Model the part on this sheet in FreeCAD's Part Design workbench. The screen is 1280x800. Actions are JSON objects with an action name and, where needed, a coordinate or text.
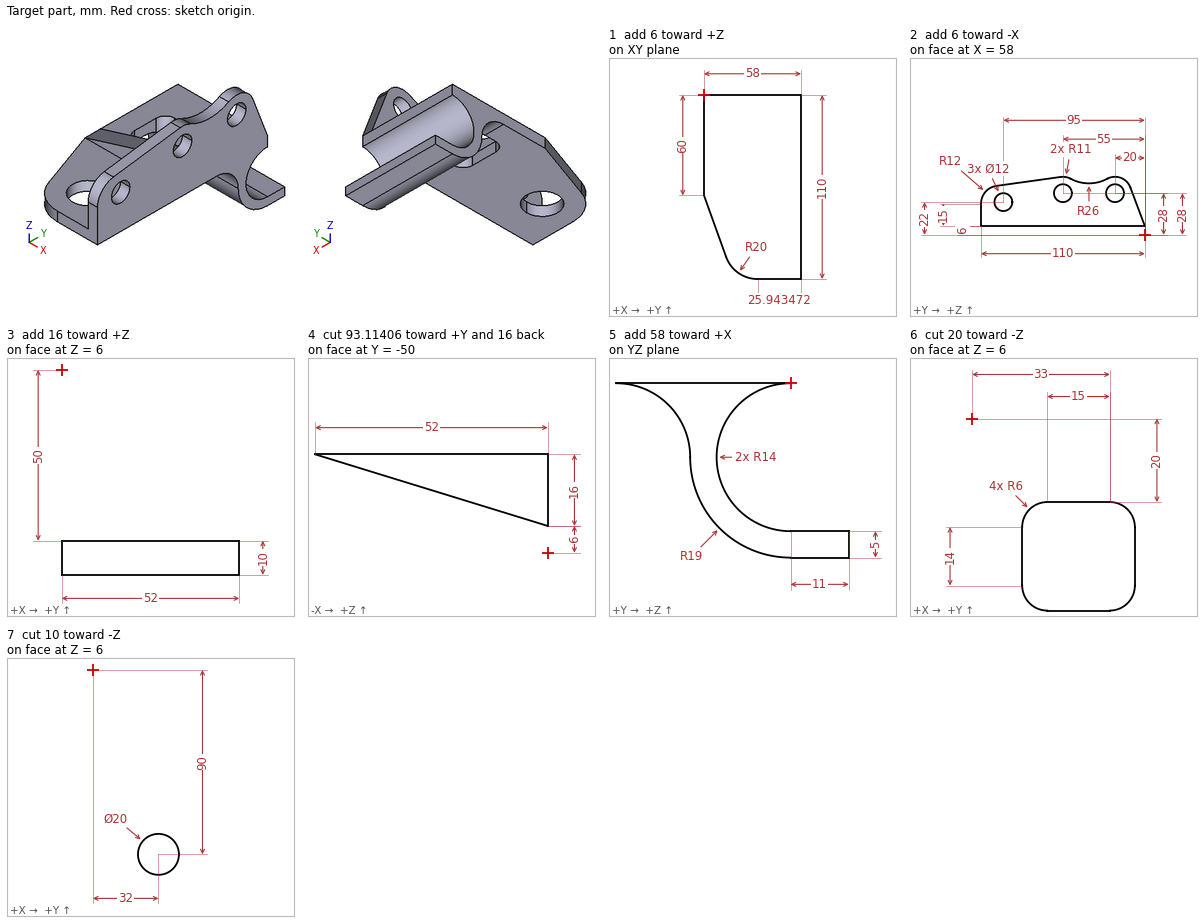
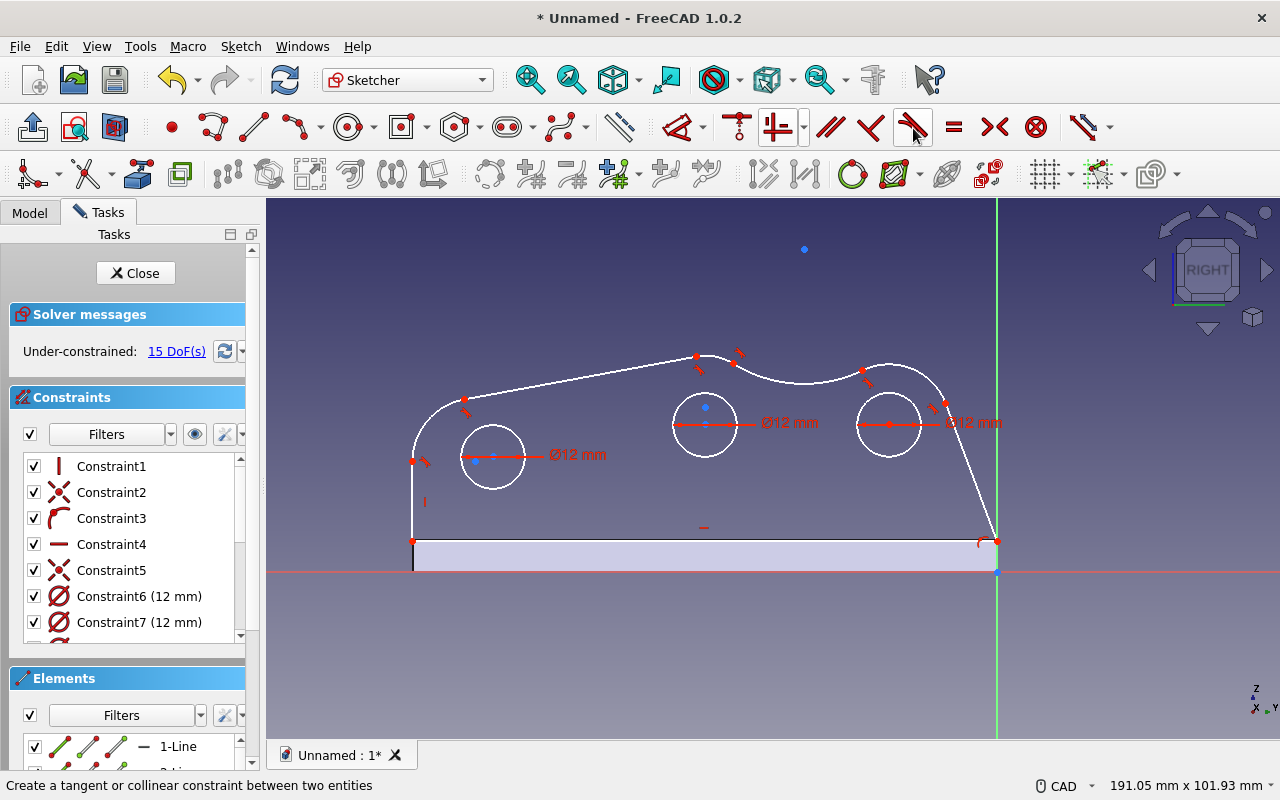
{"action": "left_click", "coordinate": [727, 402]}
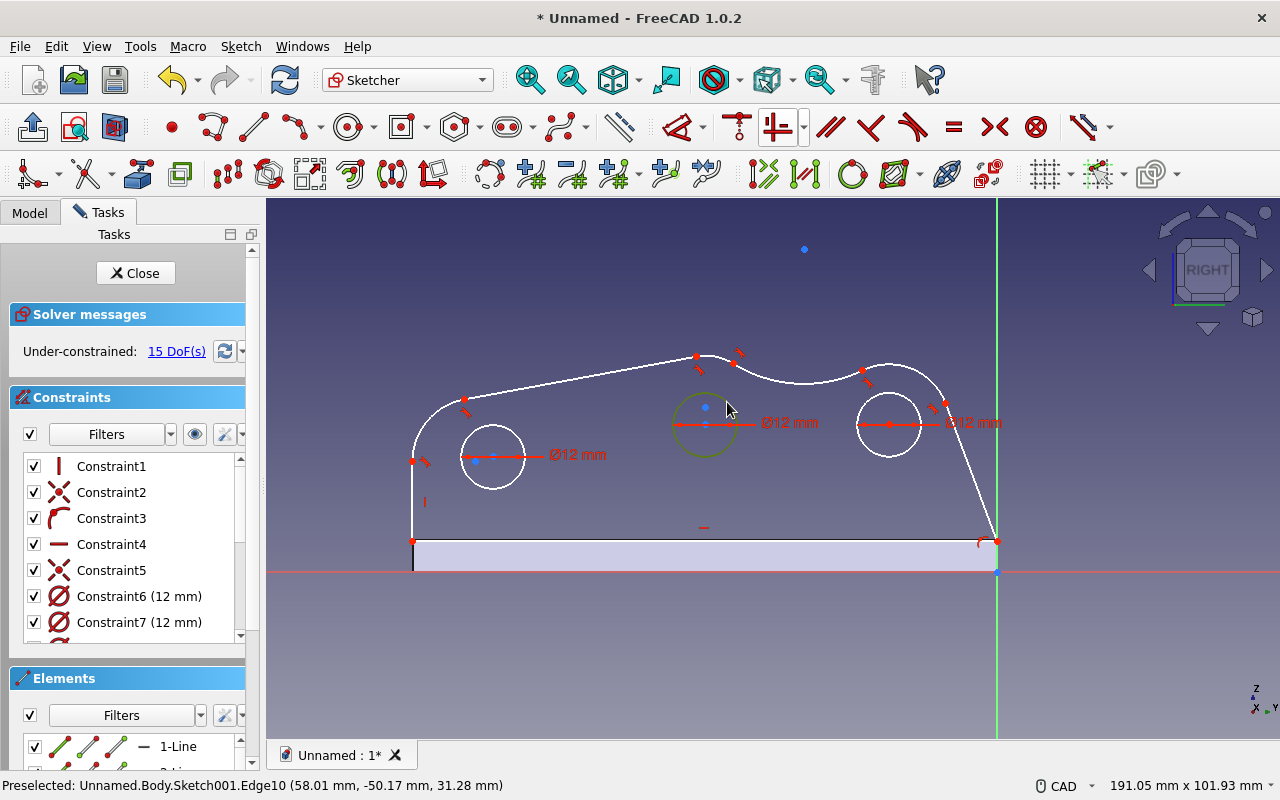
{"action": "left_click", "coordinate": [723, 359]}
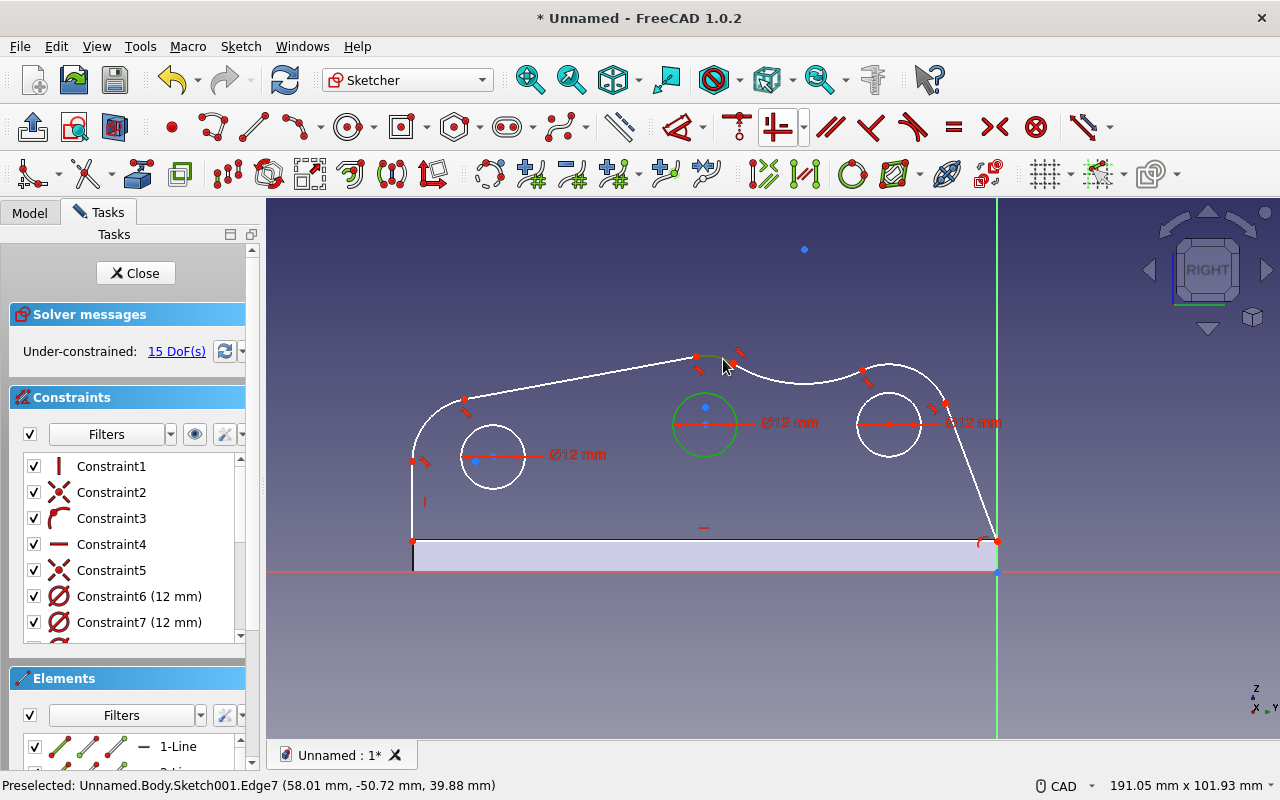
{"action": "left_click", "coordinate": [737, 128]}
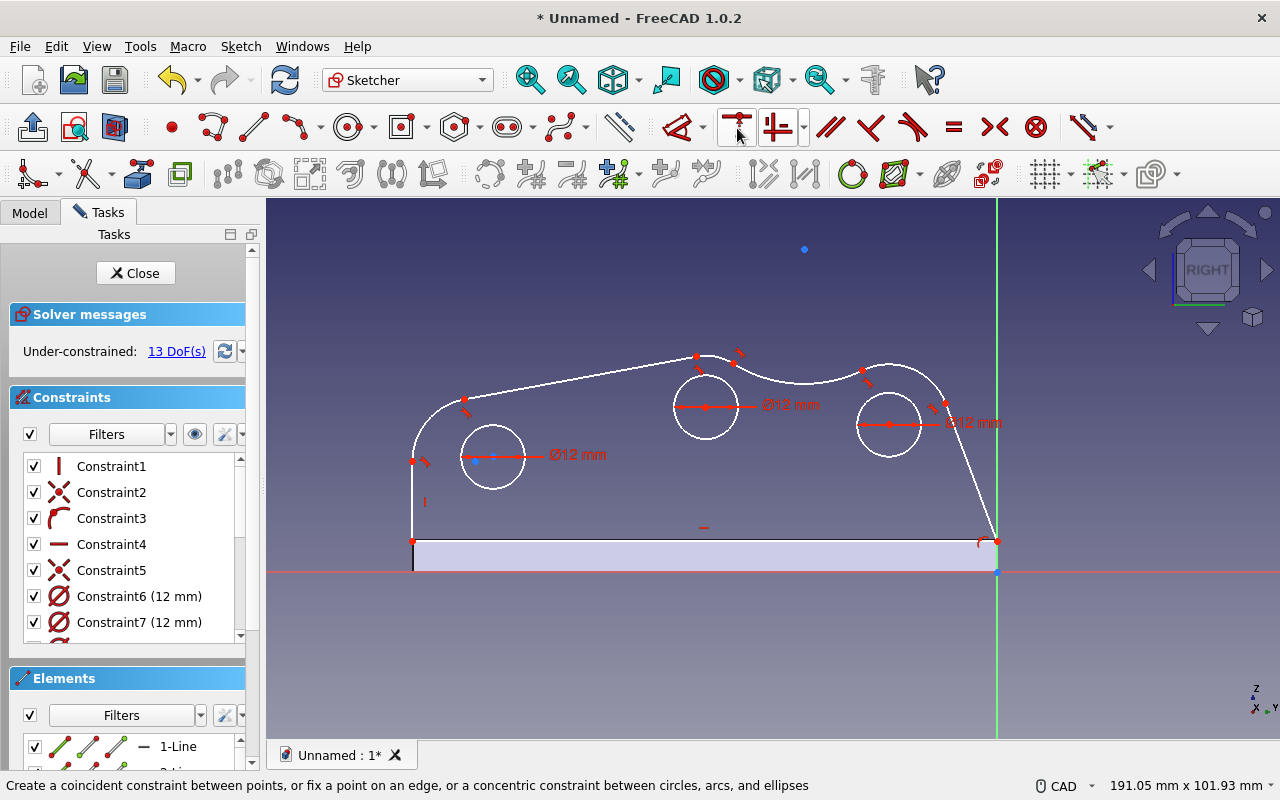
{"action": "left_click", "coordinate": [929, 379]}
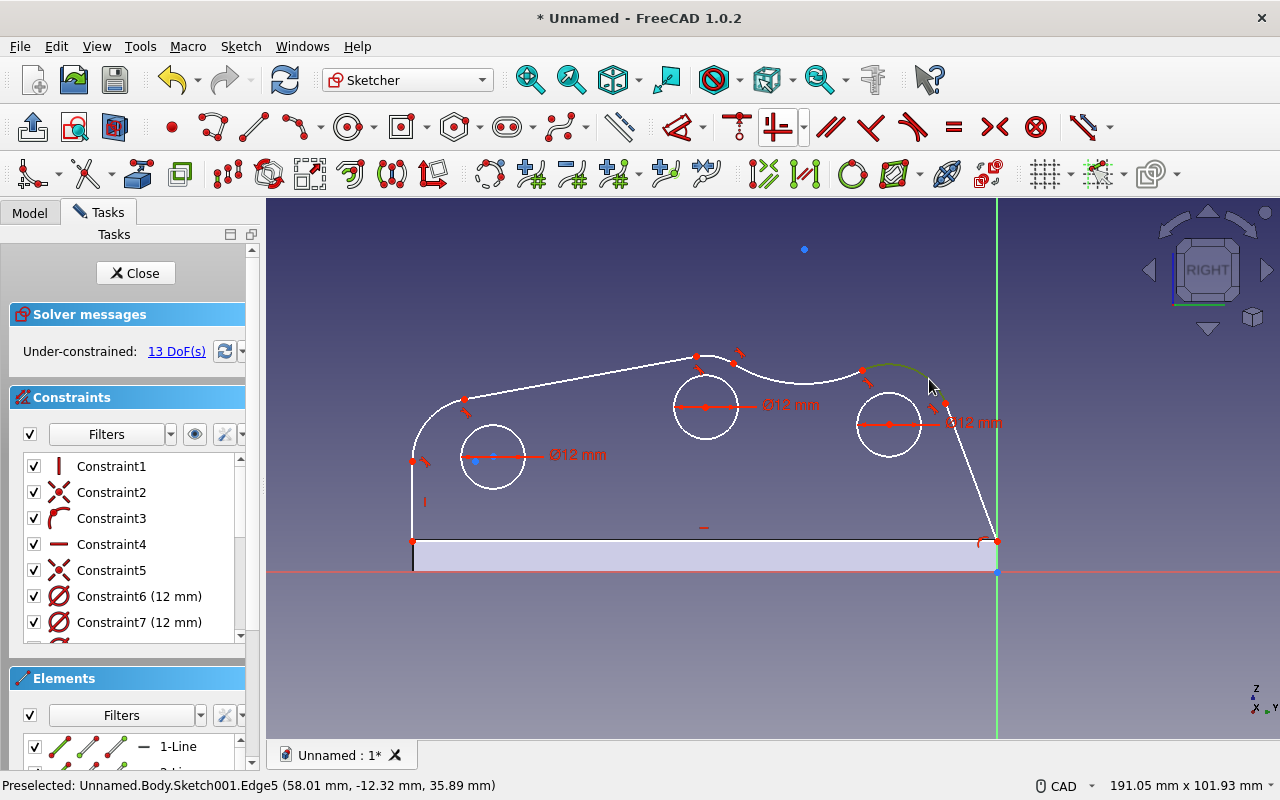
{"action": "left_click", "coordinate": [723, 359]}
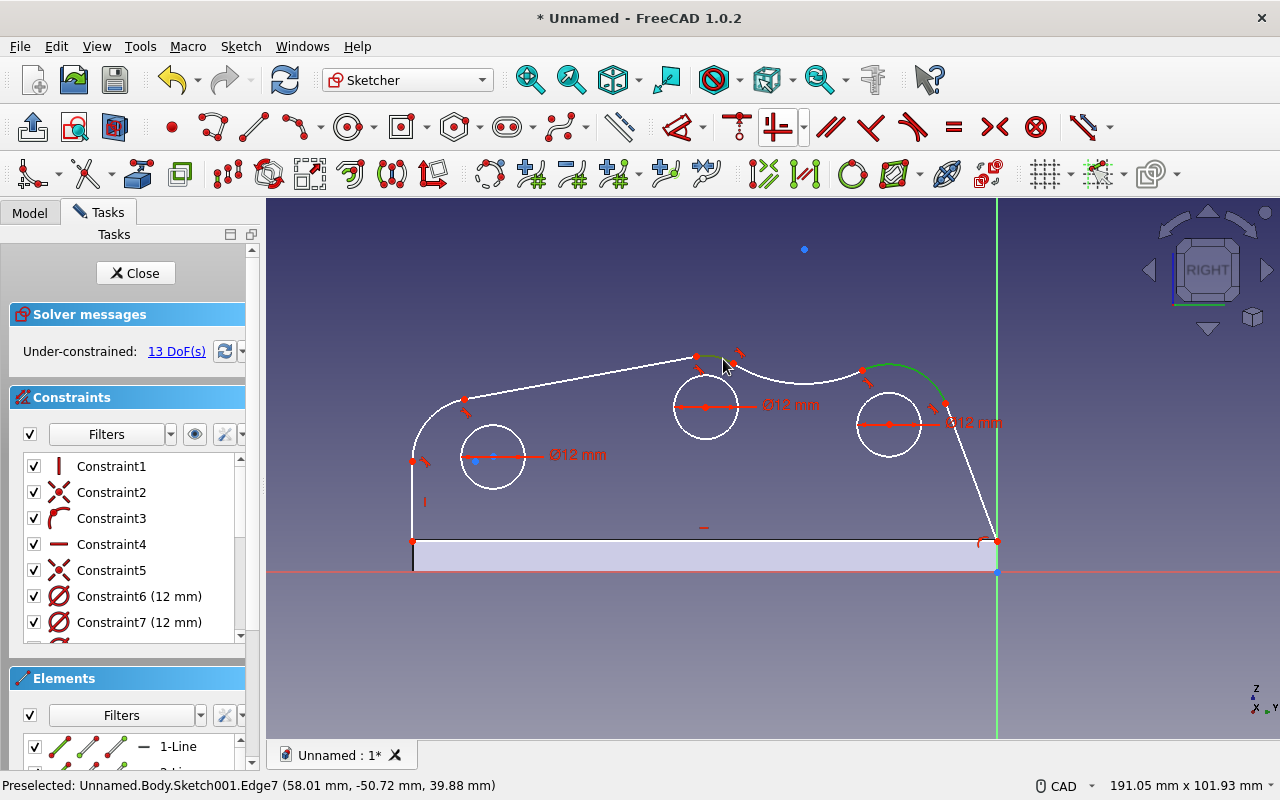
{"action": "left_click", "coordinate": [954, 128]}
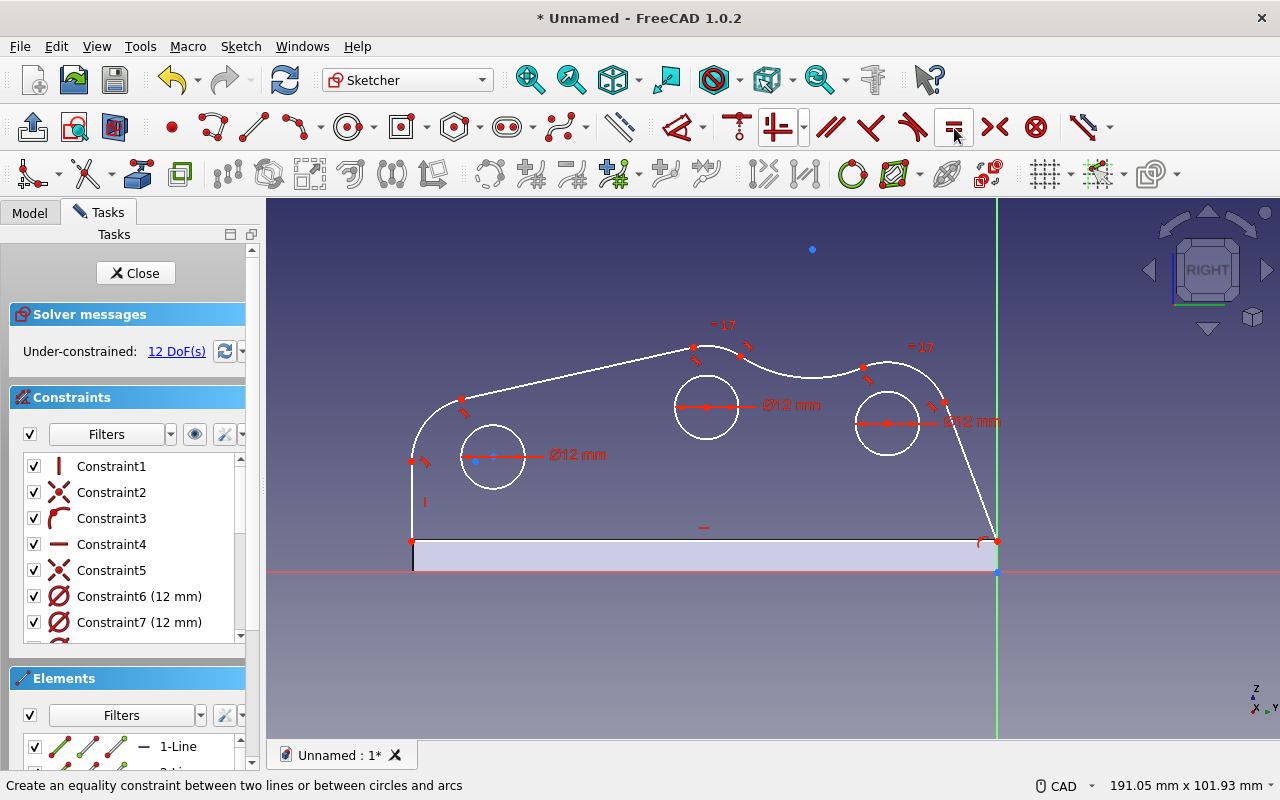
{"action": "left_click", "coordinate": [676, 128]}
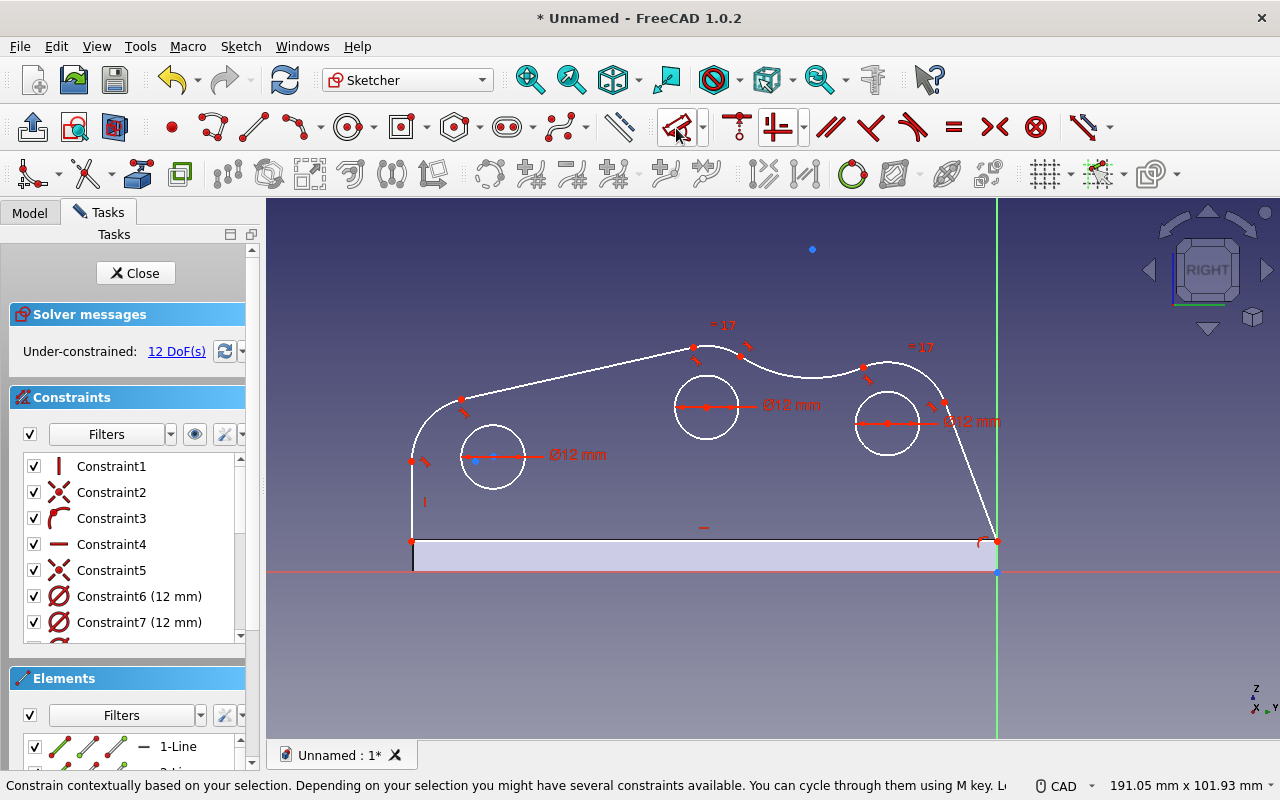
{"action": "left_click", "coordinate": [928, 378]}
{"action": "left_click", "coordinate": [949, 354]}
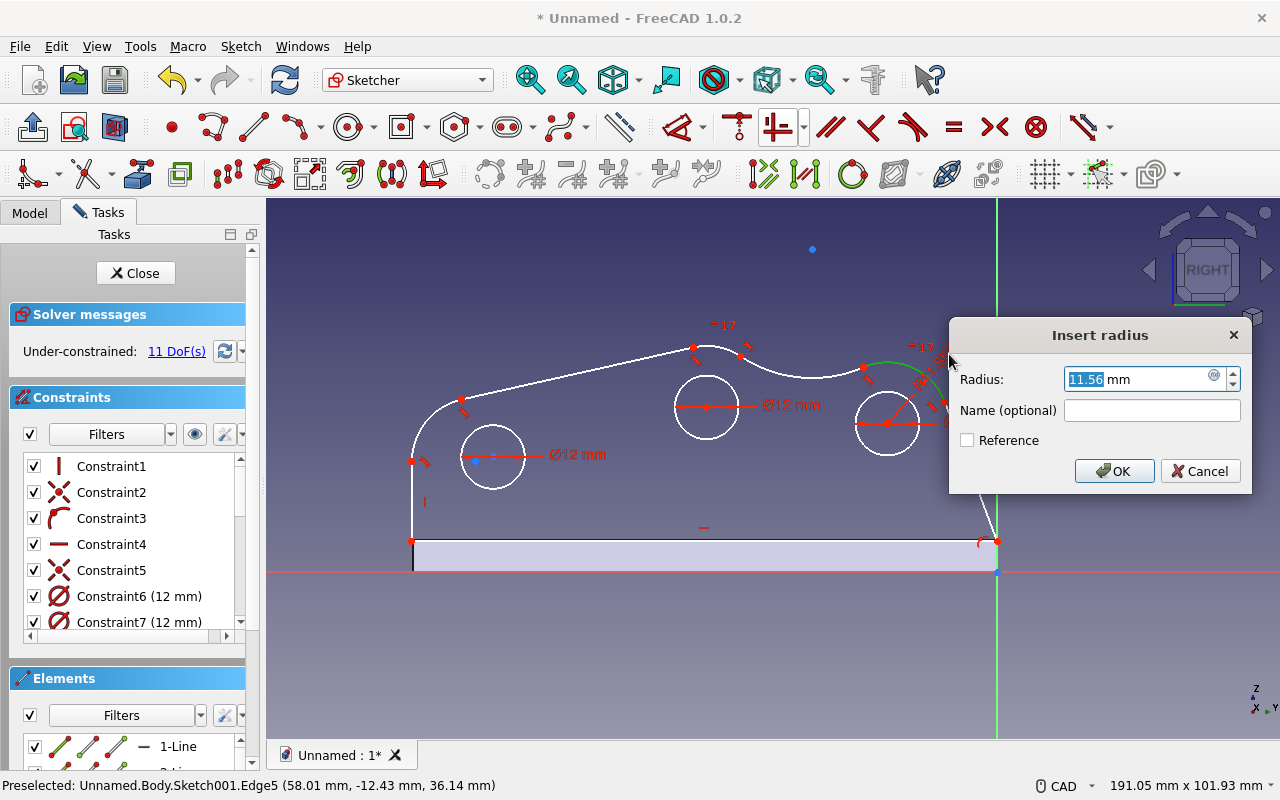
{"action": "type", "text": "11"}
{"action": "key", "text": "Return"}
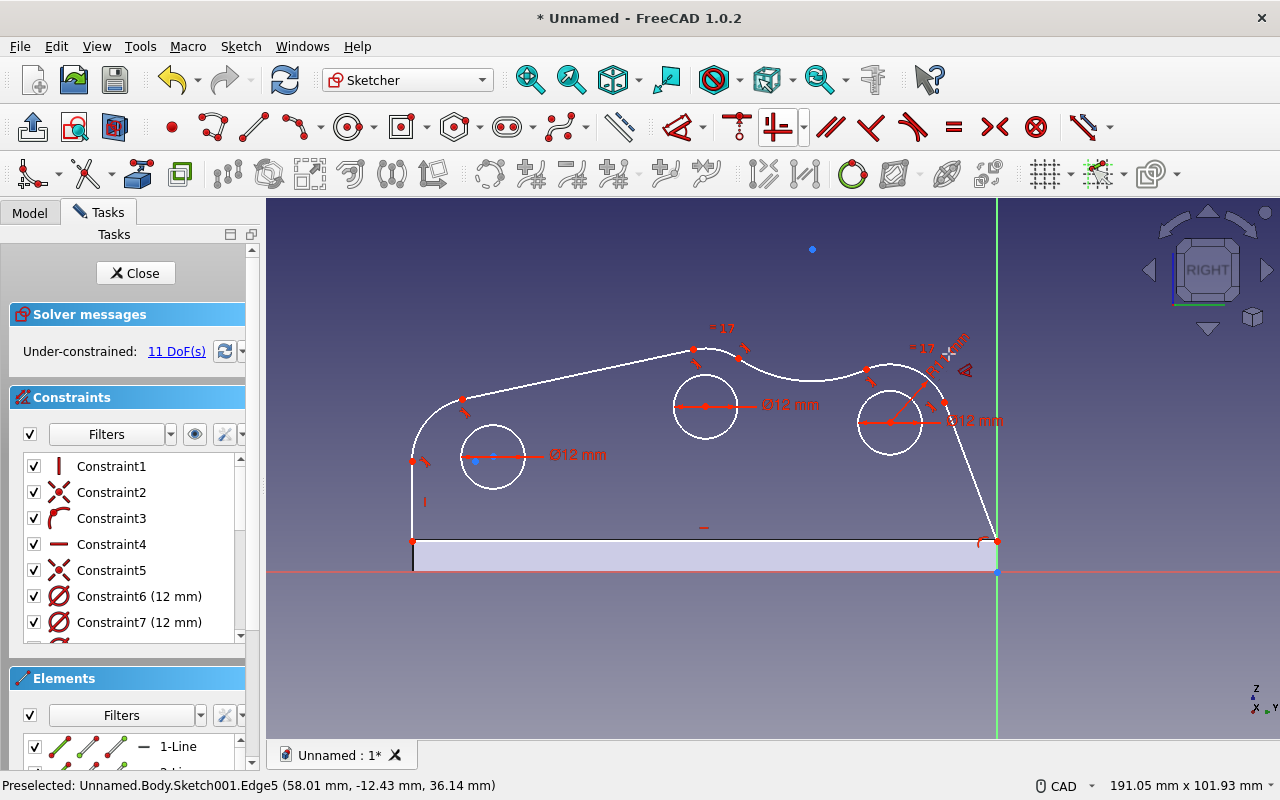
{"action": "left_click", "coordinate": [774, 376]}
{"action": "left_click", "coordinate": [765, 407]}